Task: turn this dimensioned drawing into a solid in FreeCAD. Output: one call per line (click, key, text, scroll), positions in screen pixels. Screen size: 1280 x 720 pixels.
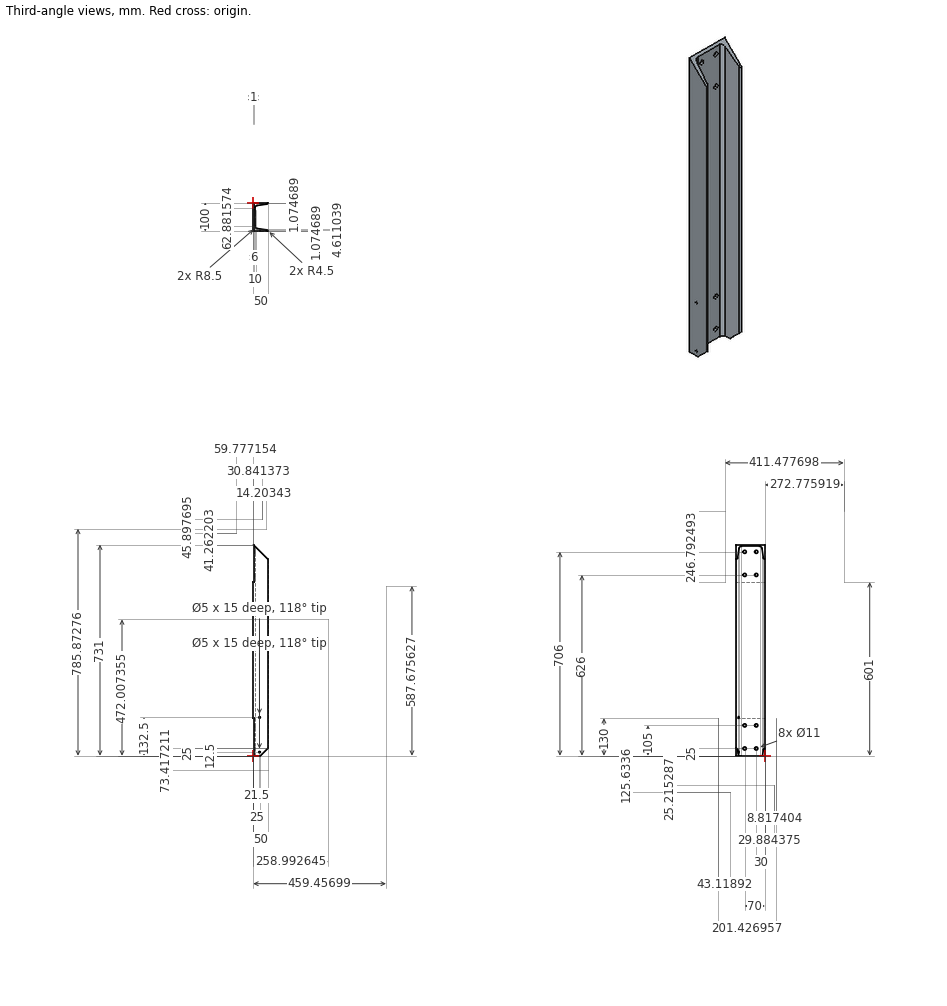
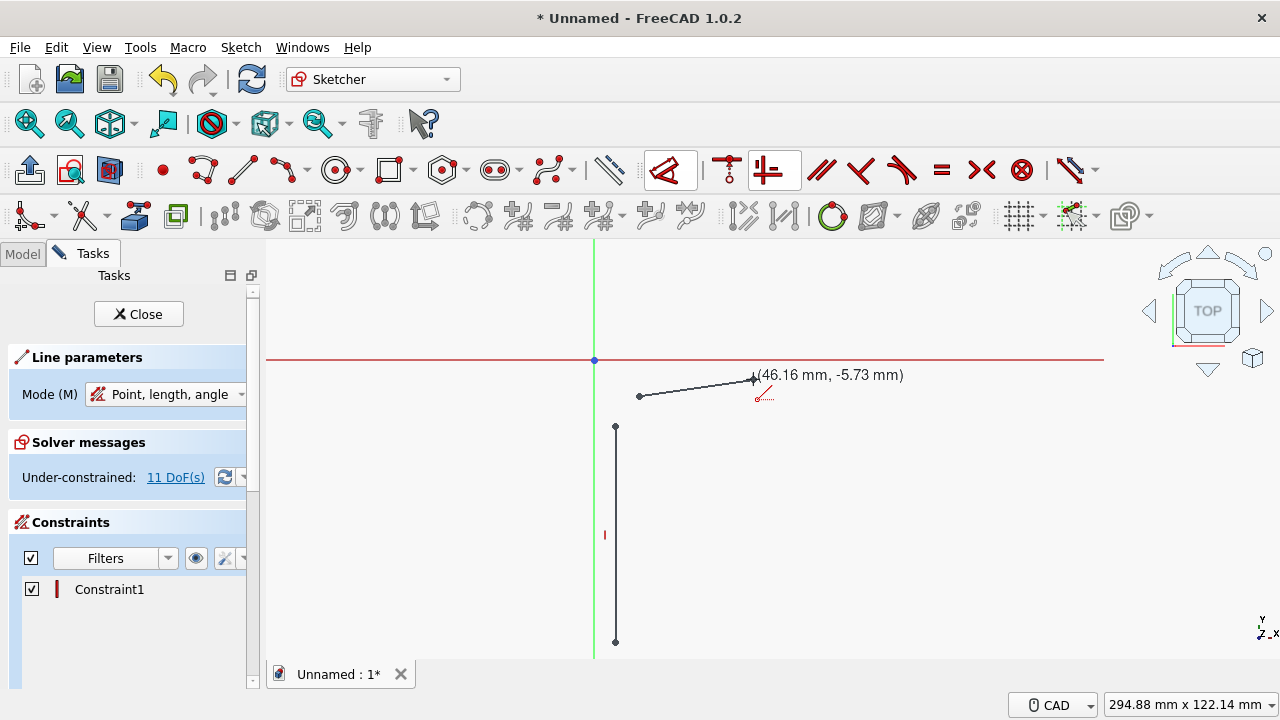
click(204, 170)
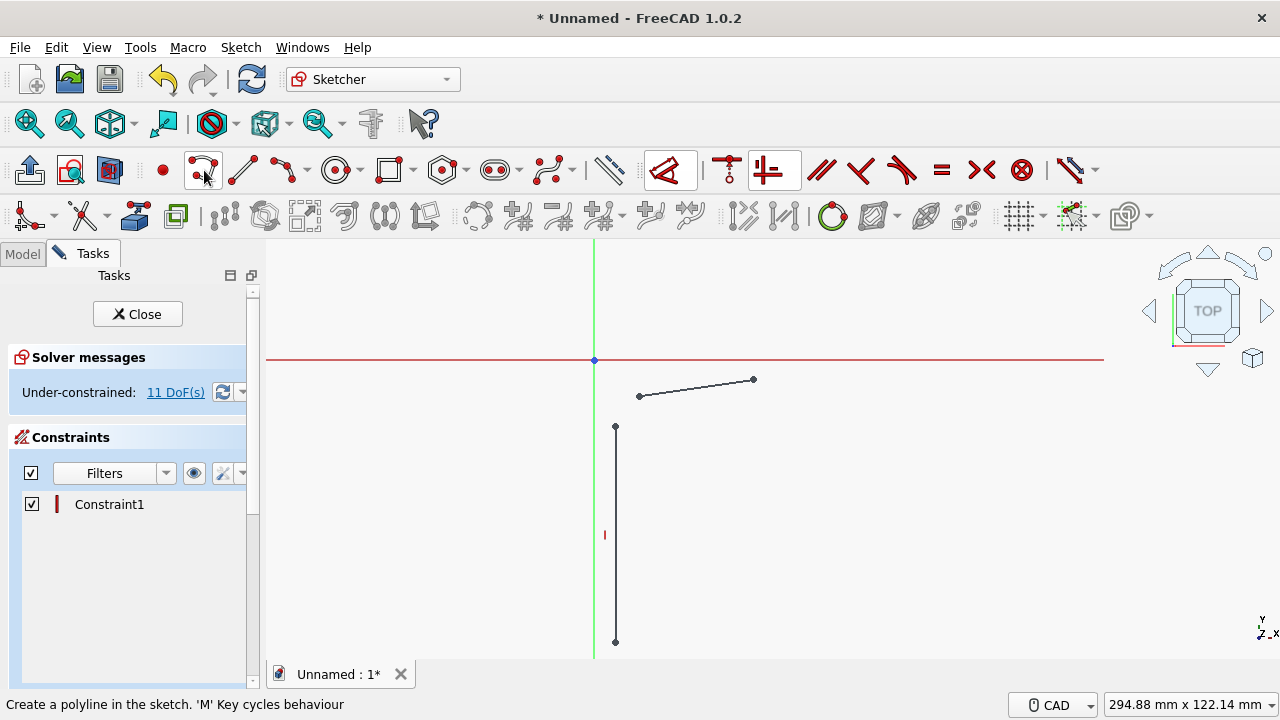
scroll(766, 364, up, 8)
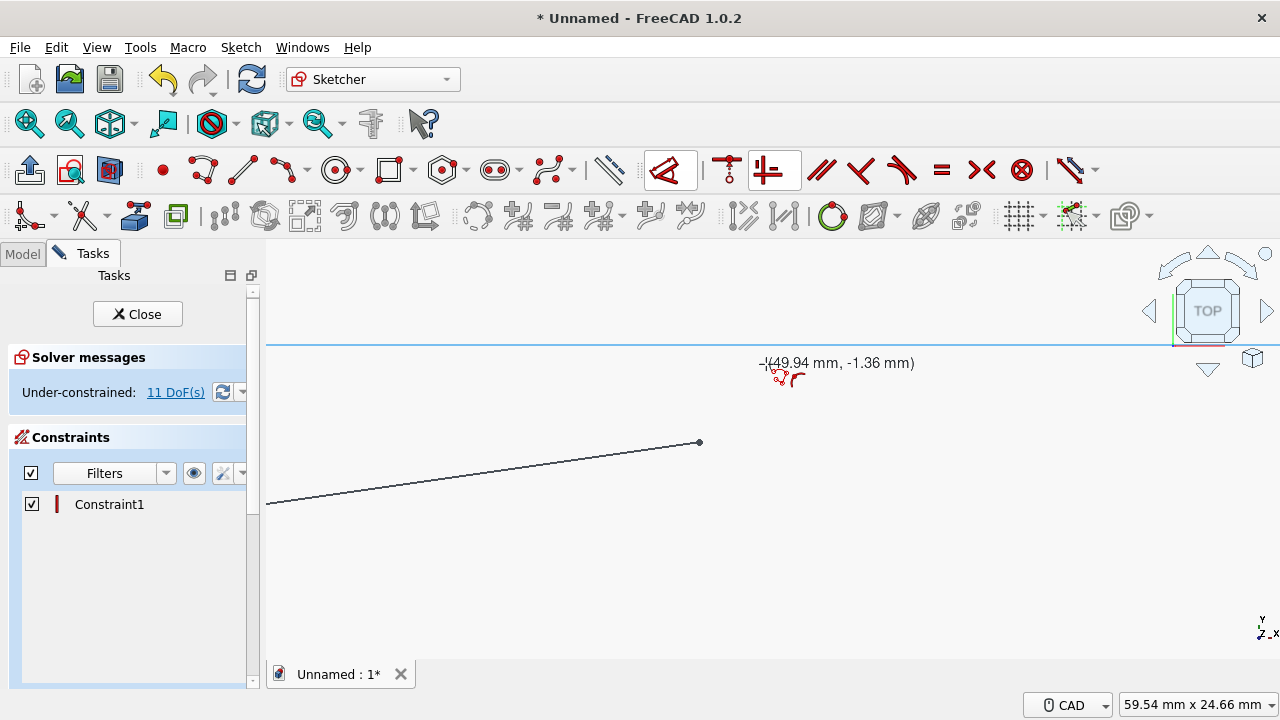
click(765, 363)
click(765, 345)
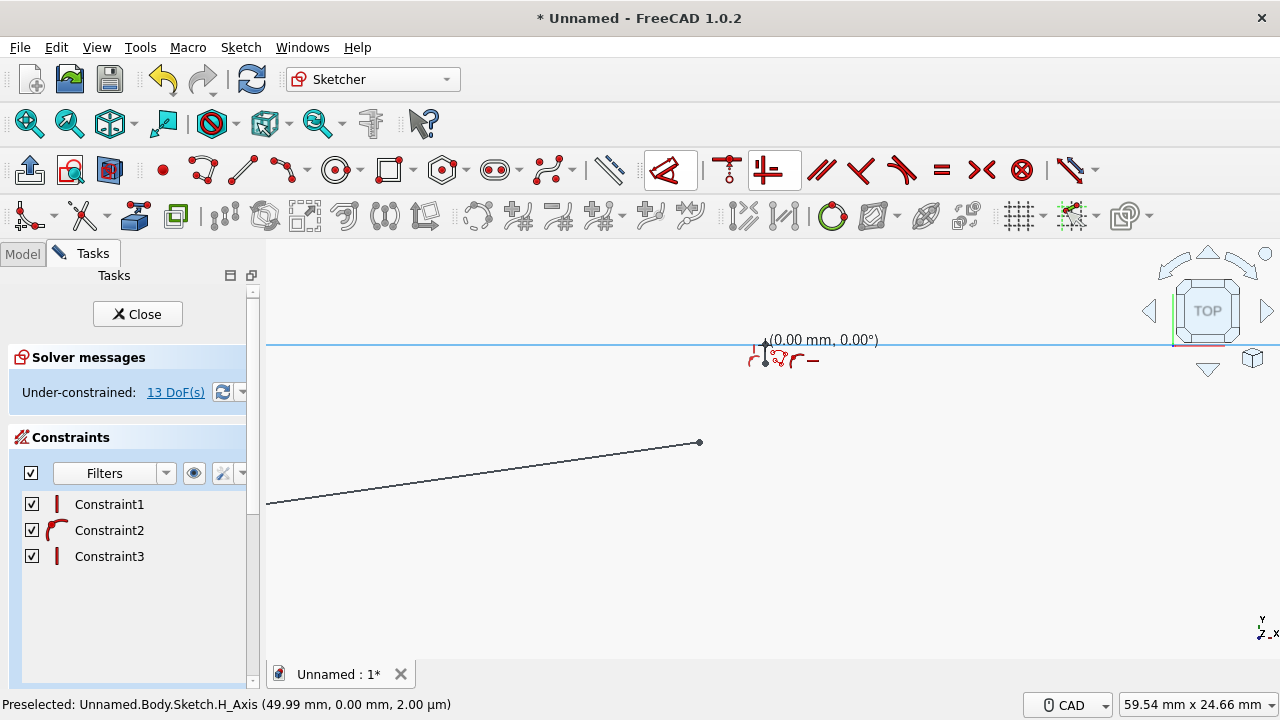
scroll(777, 301, down, 9)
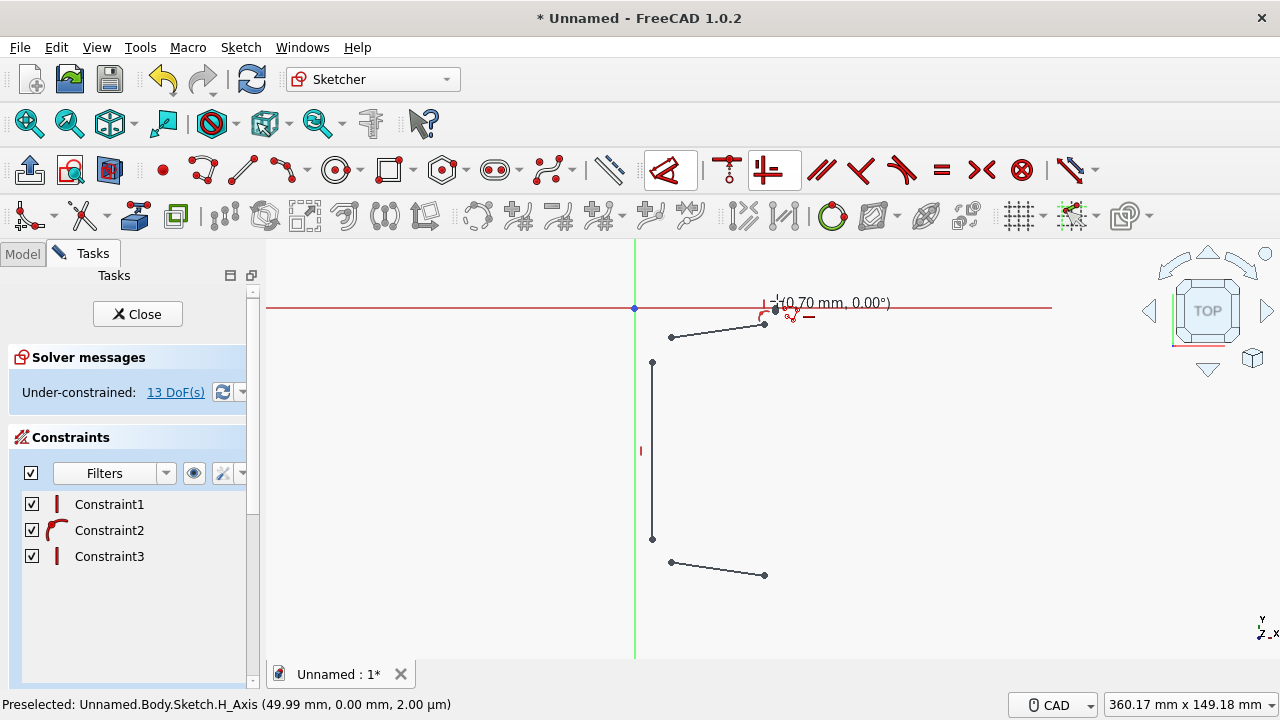
click(635, 308)
click(644, 590)
click(775, 590)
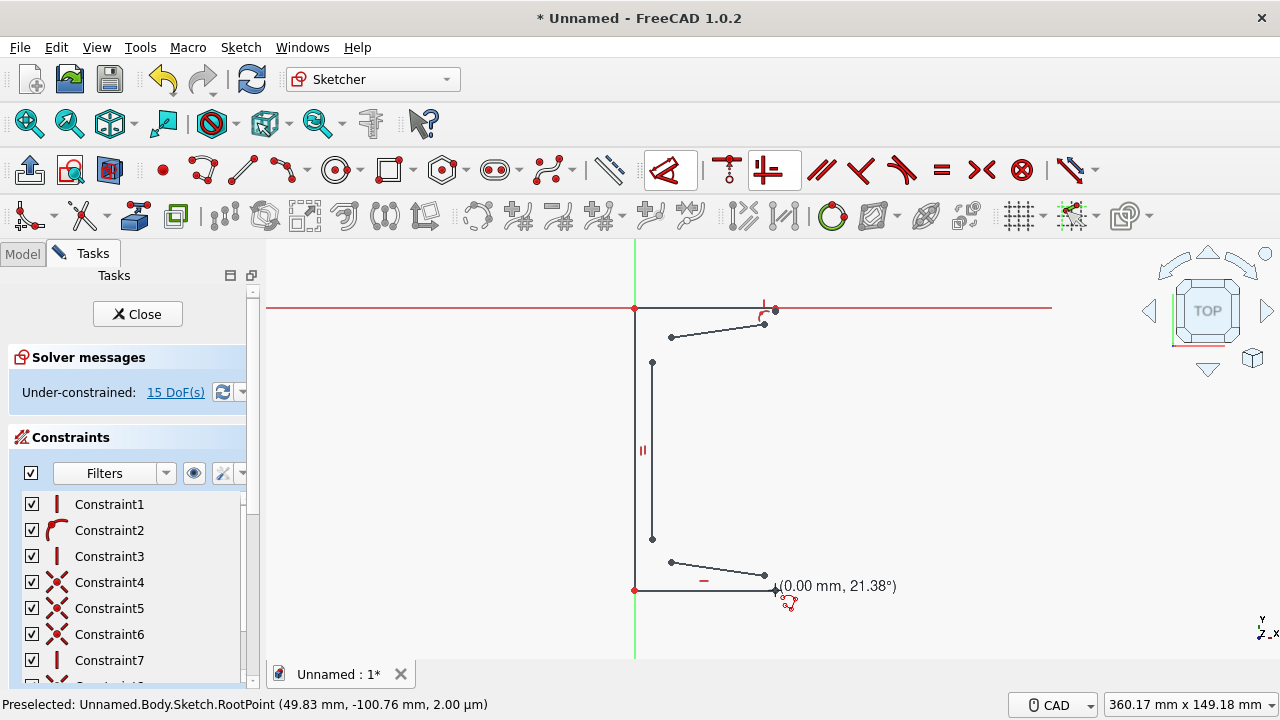
scroll(775, 587, up, 9)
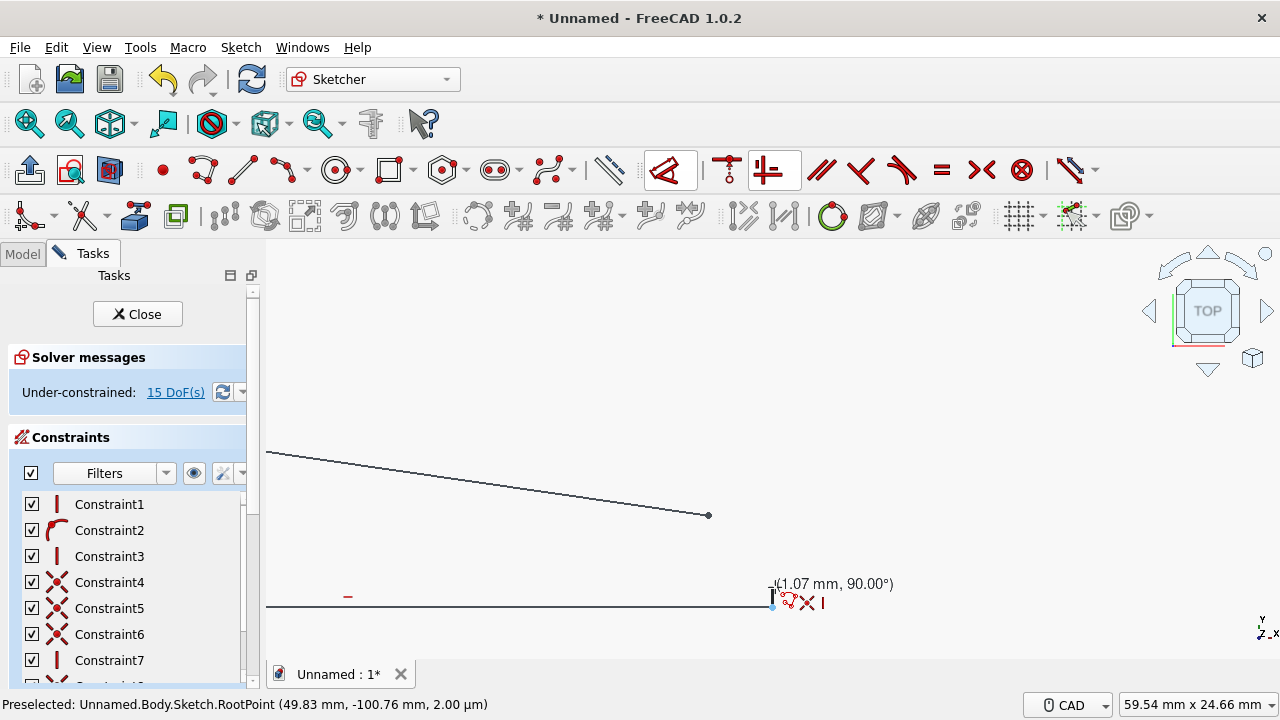
click(772, 582)
right_click(772, 582)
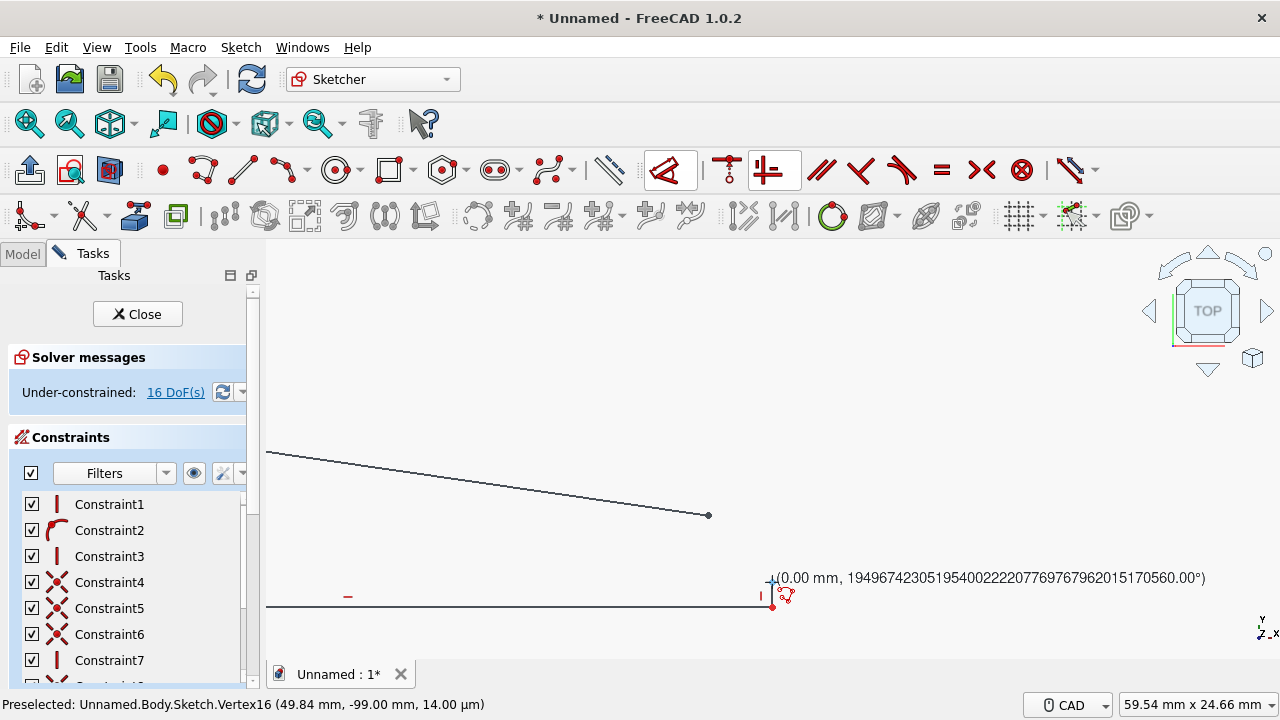
key(g)
key(3)
key(a)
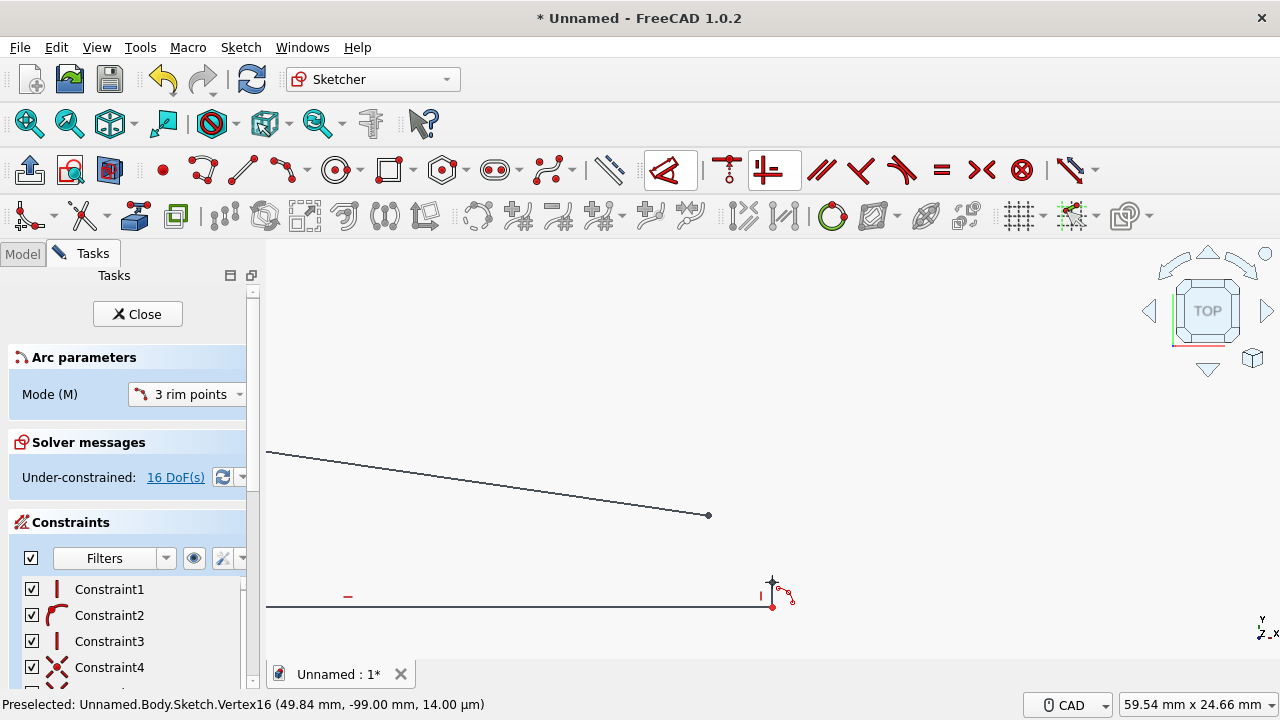
scroll(775, 588, down, 9)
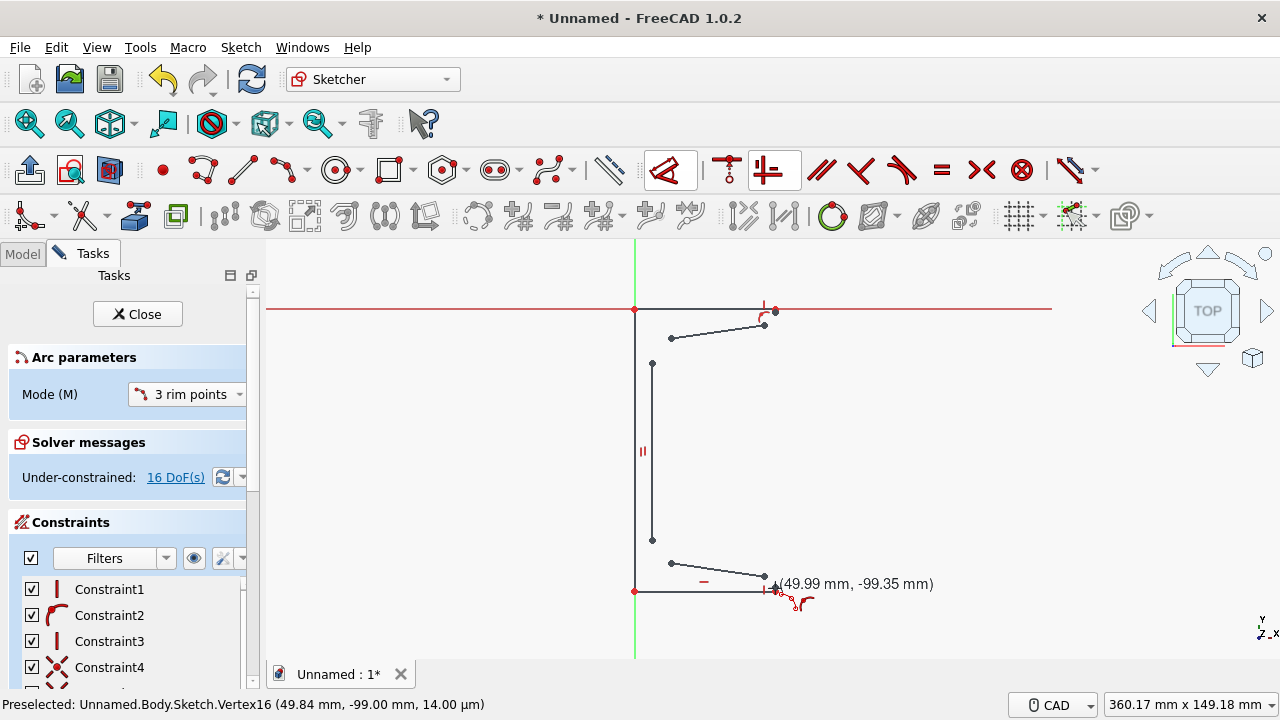
click(672, 563)
click(652, 540)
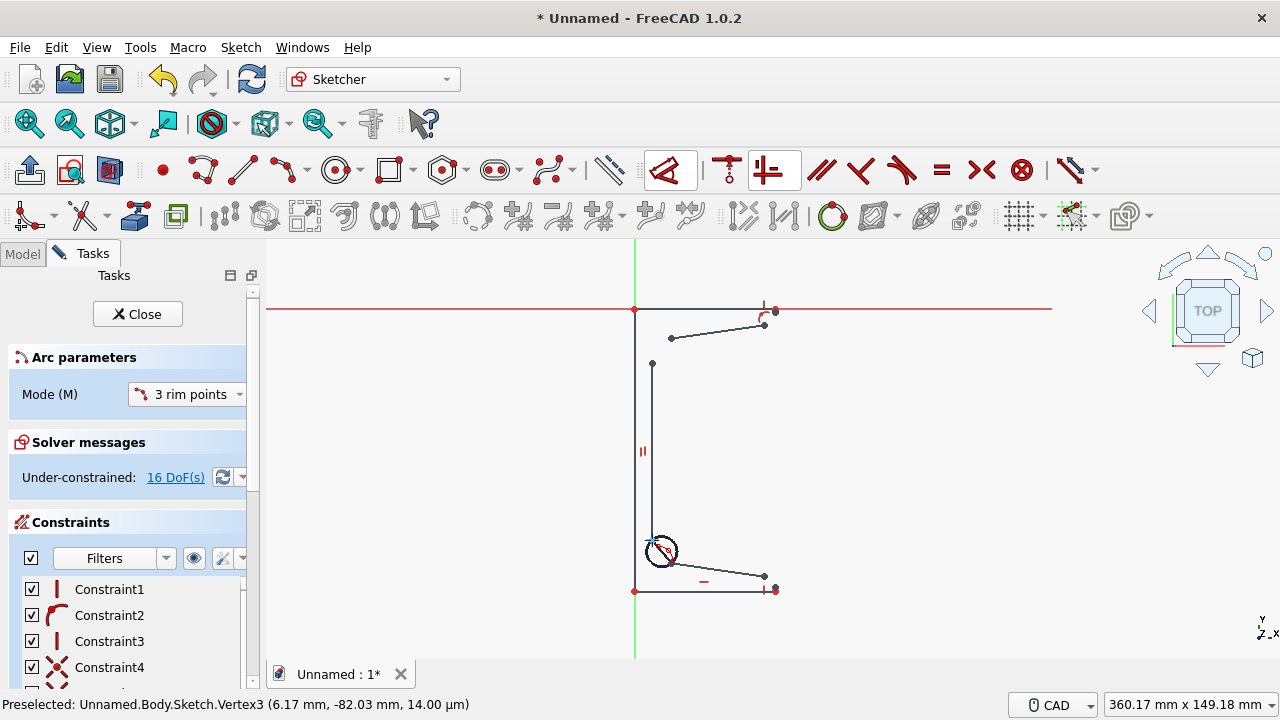
scroll(657, 554, up, 5)